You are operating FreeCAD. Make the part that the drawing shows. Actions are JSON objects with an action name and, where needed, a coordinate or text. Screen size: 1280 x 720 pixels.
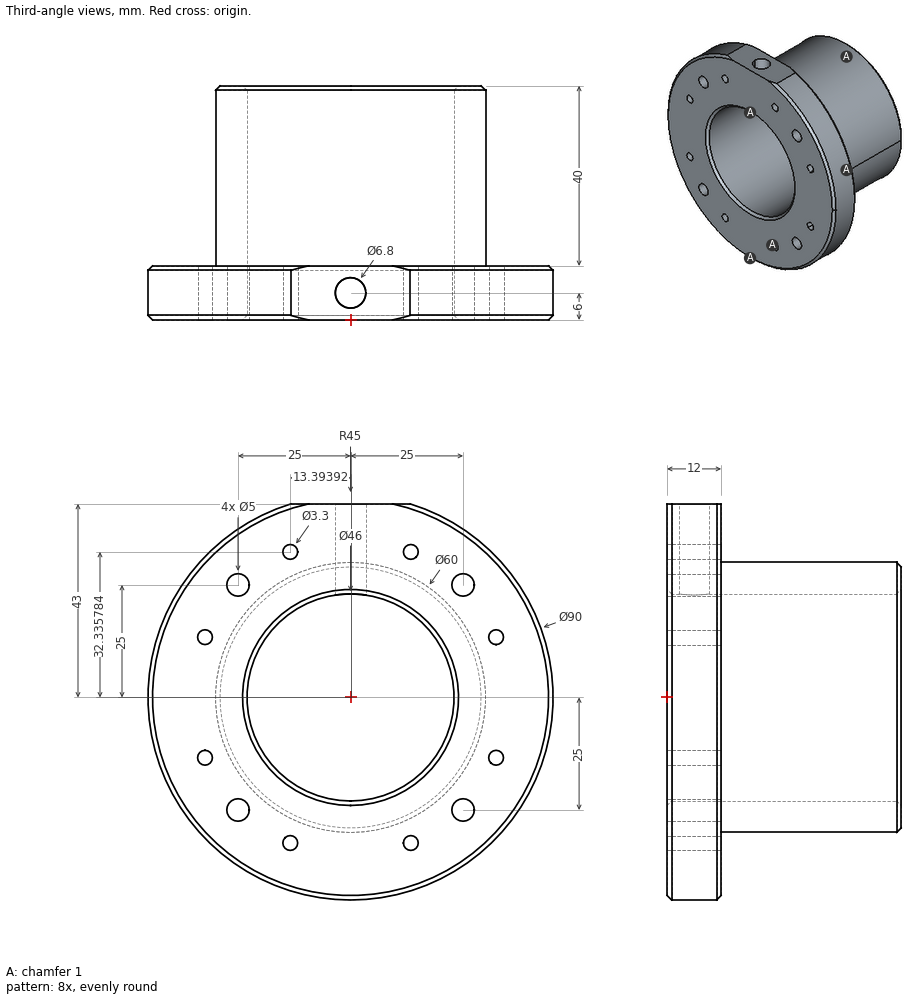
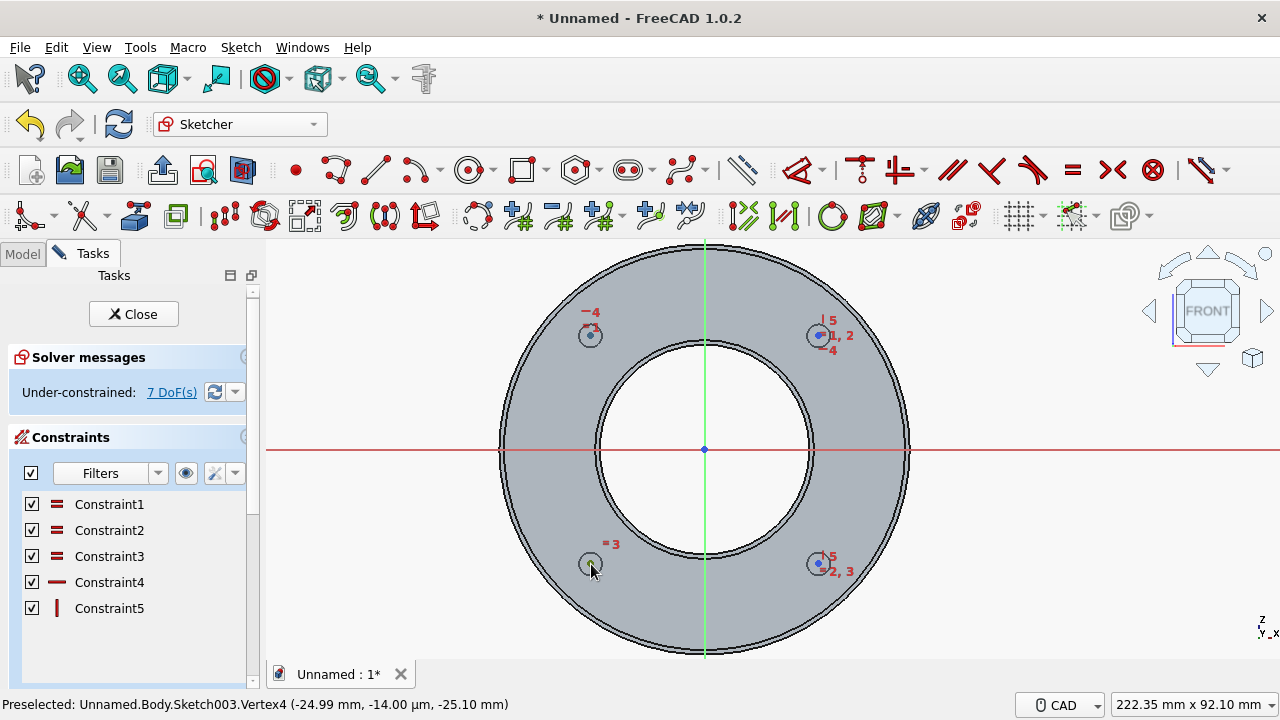
{"action": "key", "text": "v"}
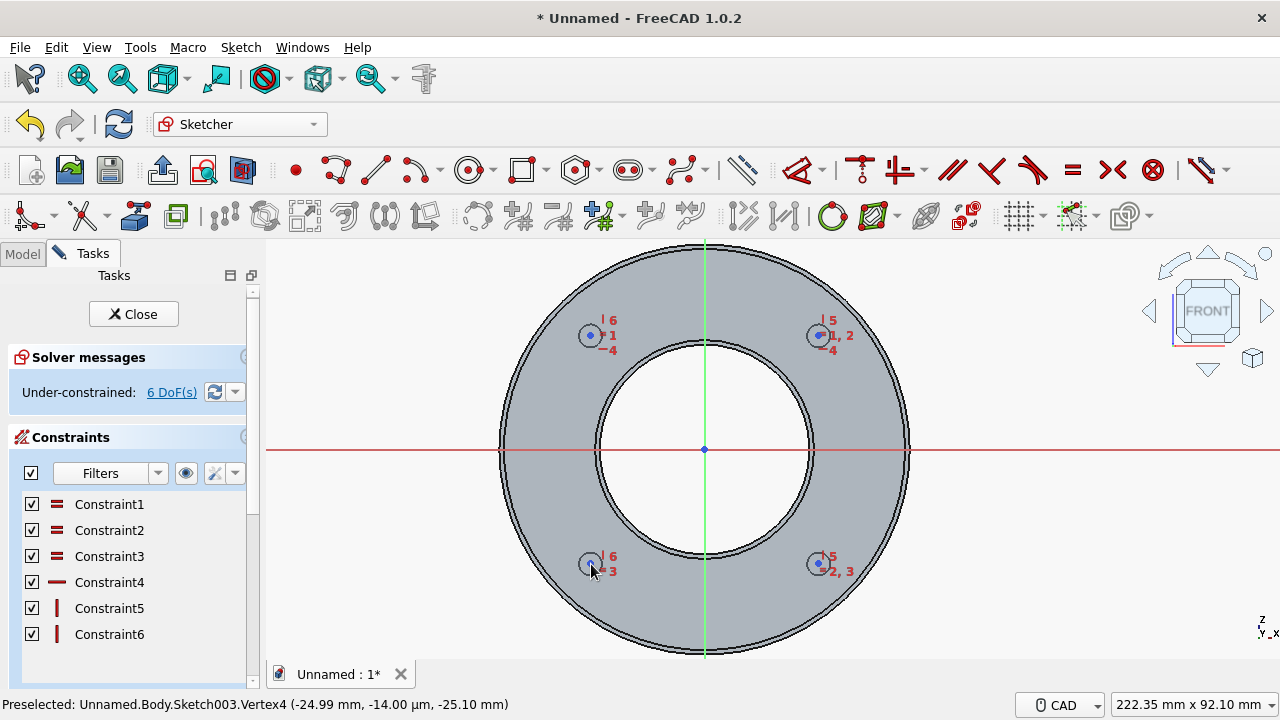
{"action": "scroll", "coordinate": [819, 564], "scroll_direction": "up", "scroll_amount": 4}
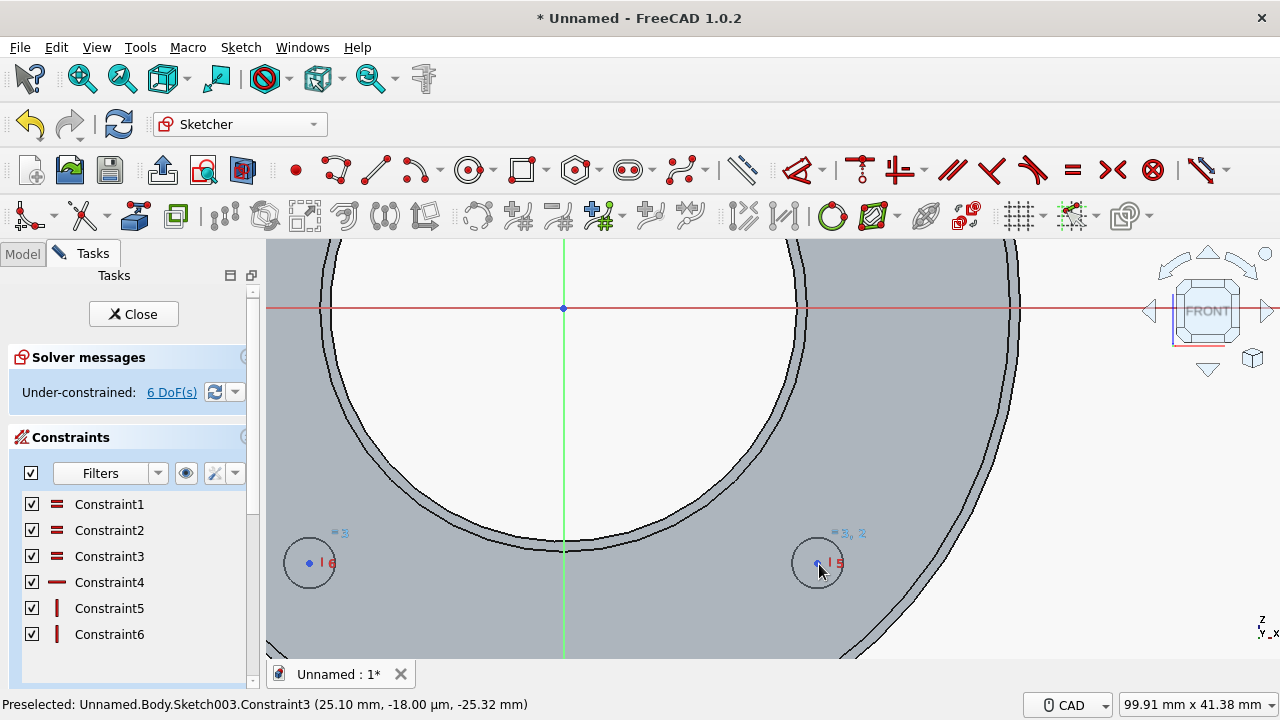
{"action": "left_click", "coordinate": [818, 563]}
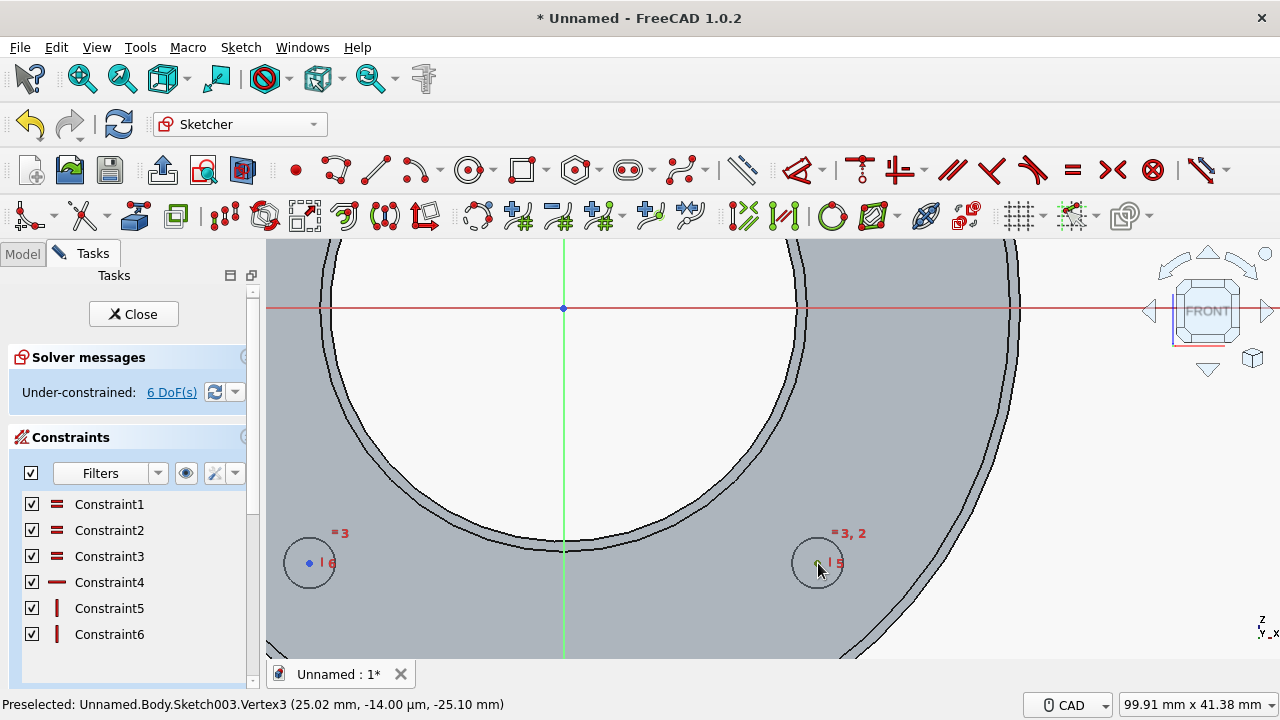
{"action": "left_click", "coordinate": [310, 563]}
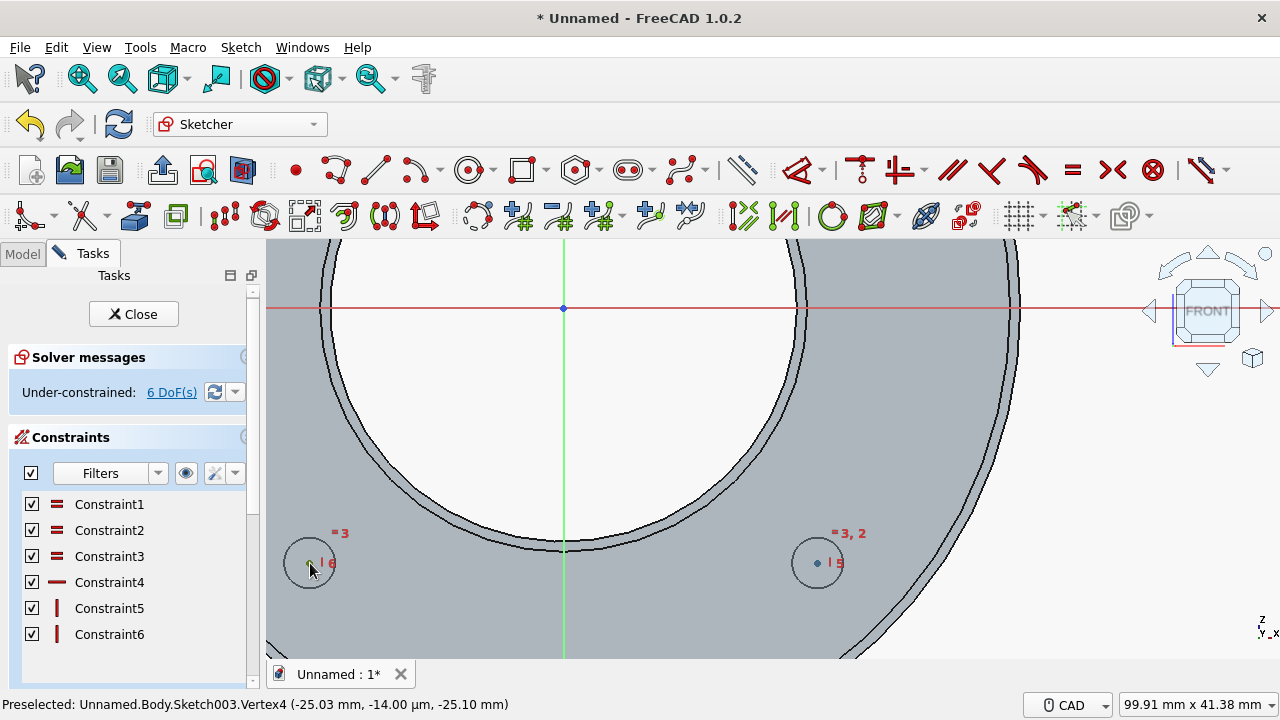
{"action": "key", "text": "h"}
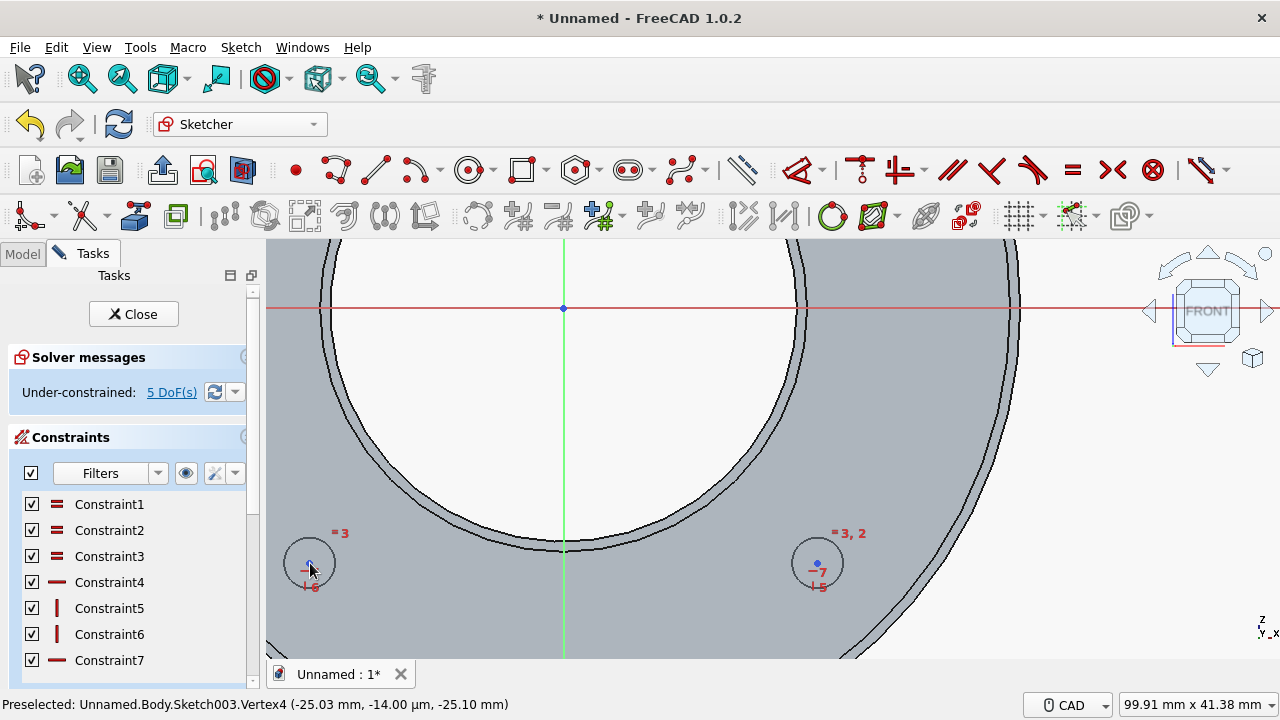
{"action": "left_click", "coordinate": [798, 170]}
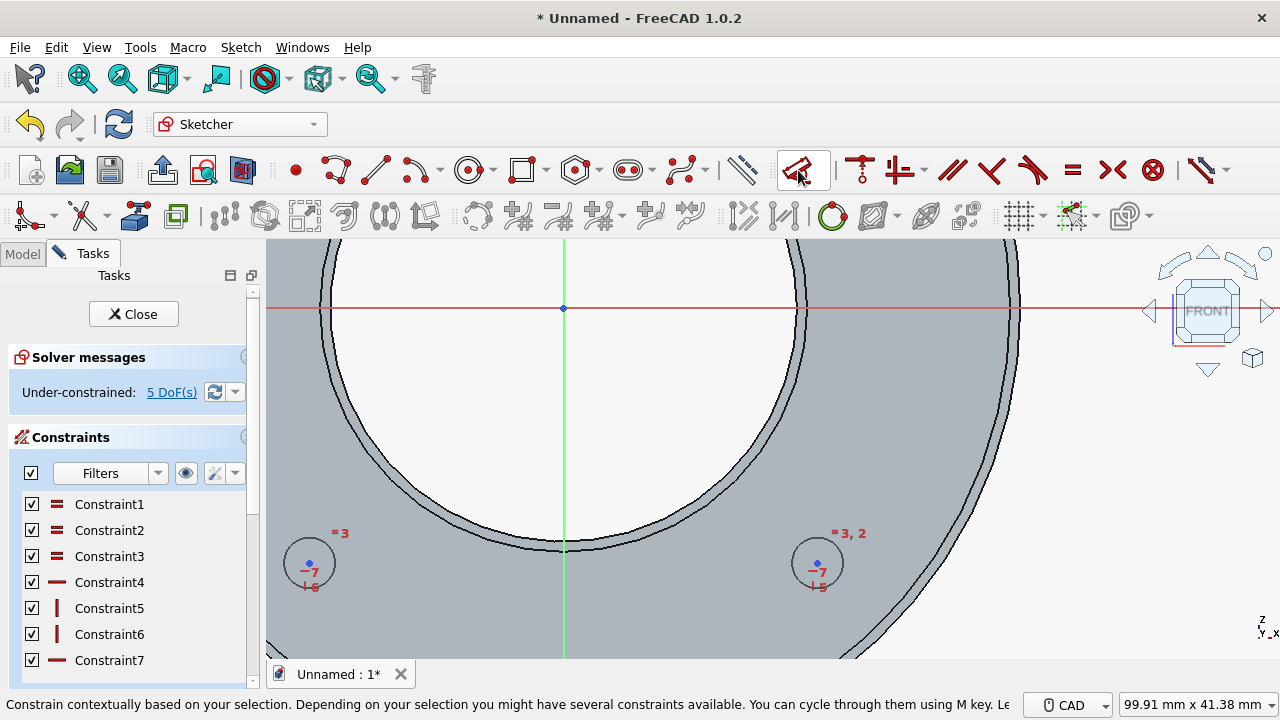
{"action": "scroll", "coordinate": [819, 564], "scroll_direction": "down", "scroll_amount": 4}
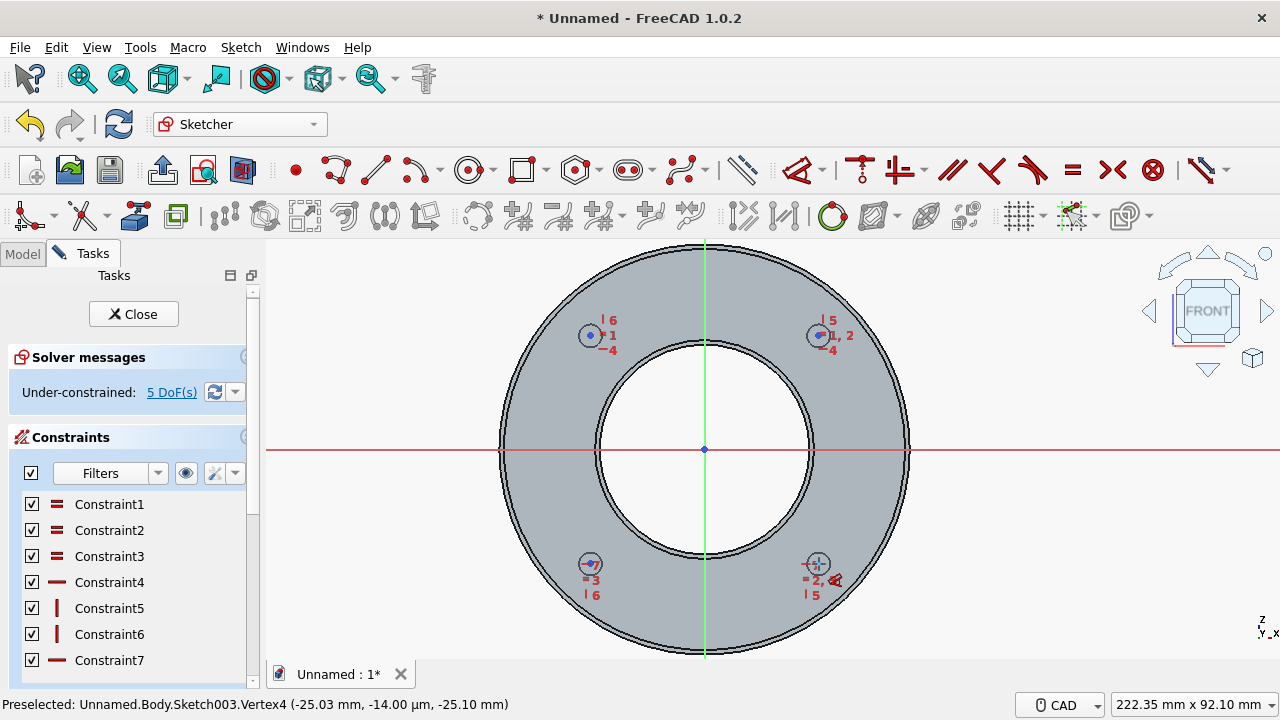
{"action": "scroll", "coordinate": [598, 328], "scroll_direction": "up", "scroll_amount": 3}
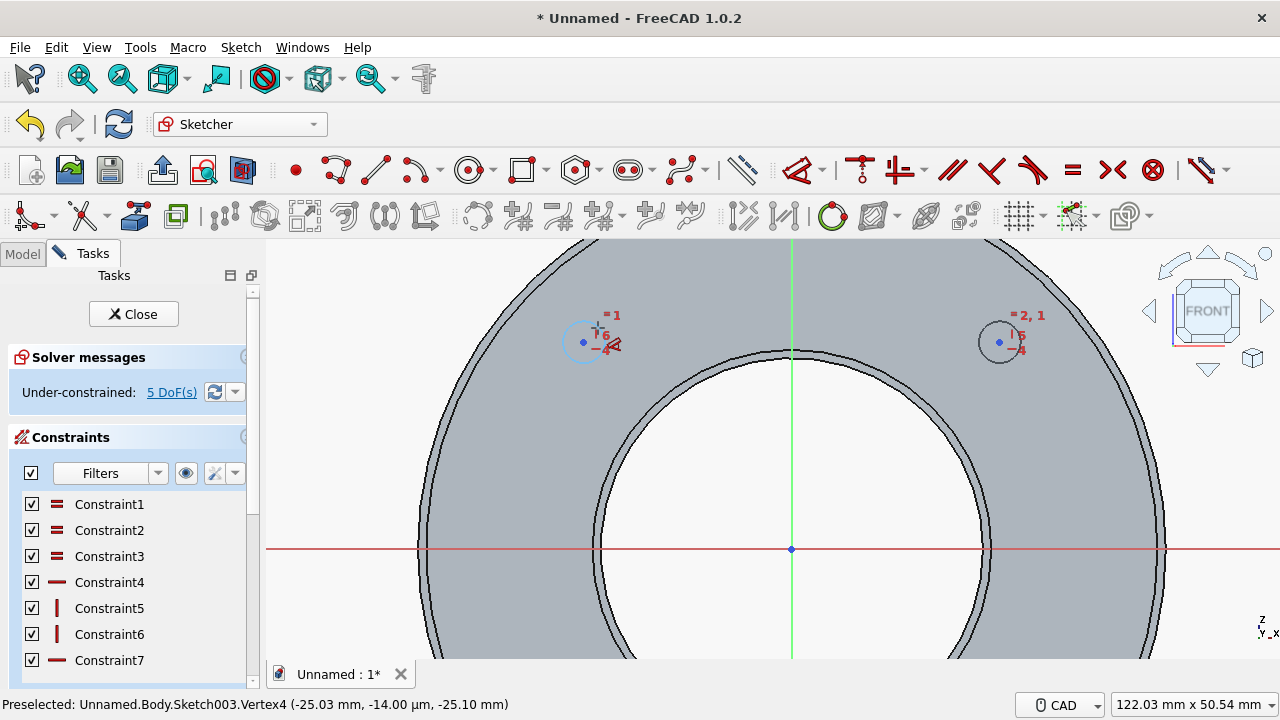
{"action": "left_click", "coordinate": [599, 327]}
{"action": "left_click", "coordinate": [622, 304]}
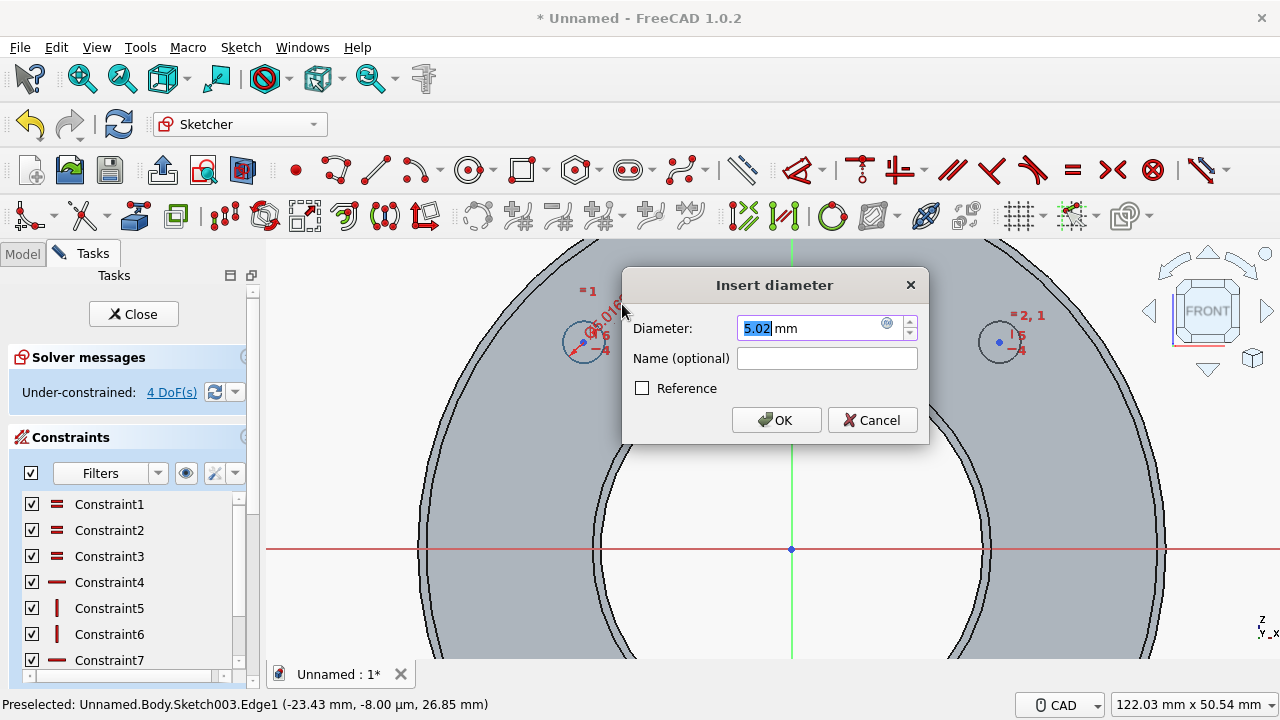
{"action": "type", "text": "5"}
{"action": "key", "text": "Return"}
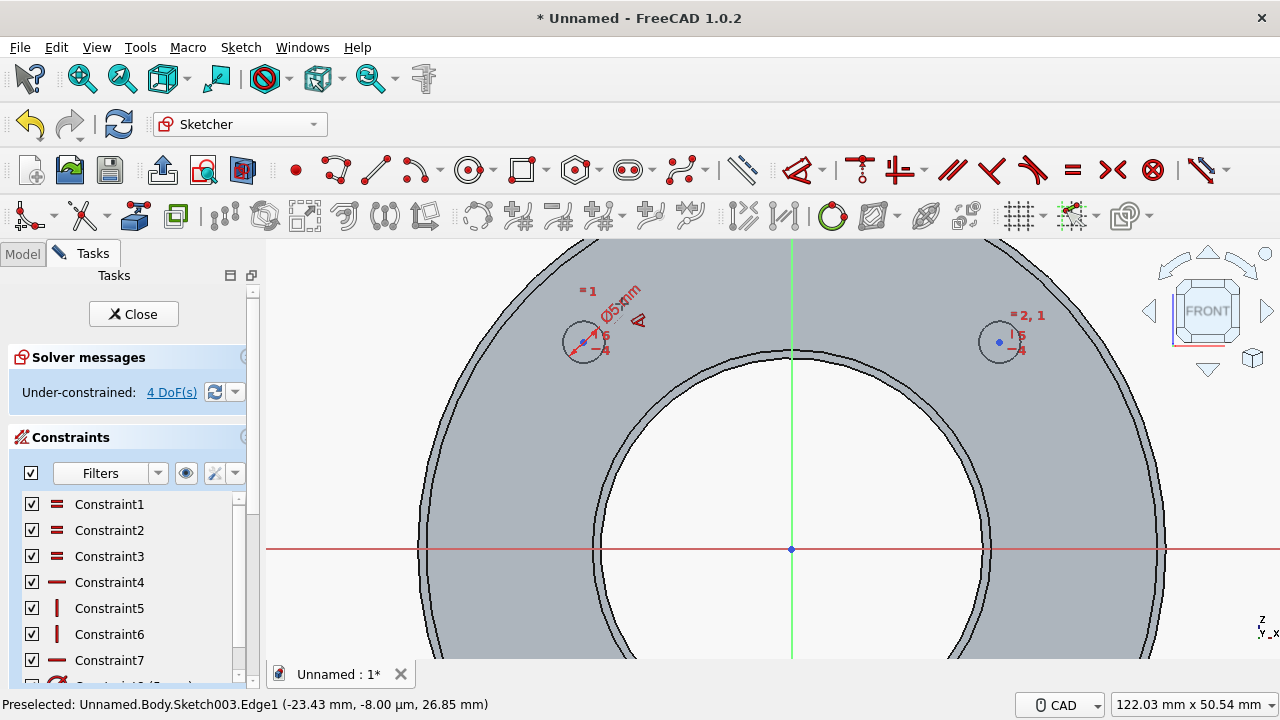
{"action": "left_click", "coordinate": [584, 342]}
{"action": "left_click", "coordinate": [736, 308]}